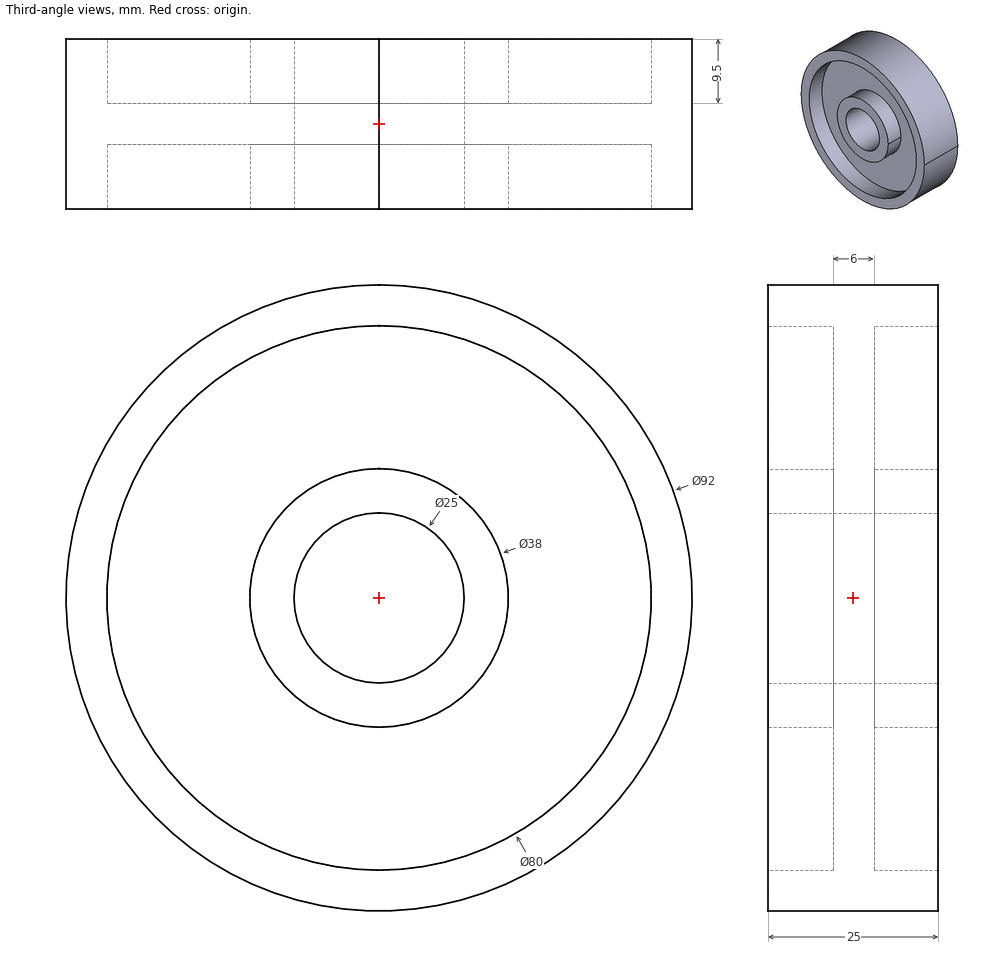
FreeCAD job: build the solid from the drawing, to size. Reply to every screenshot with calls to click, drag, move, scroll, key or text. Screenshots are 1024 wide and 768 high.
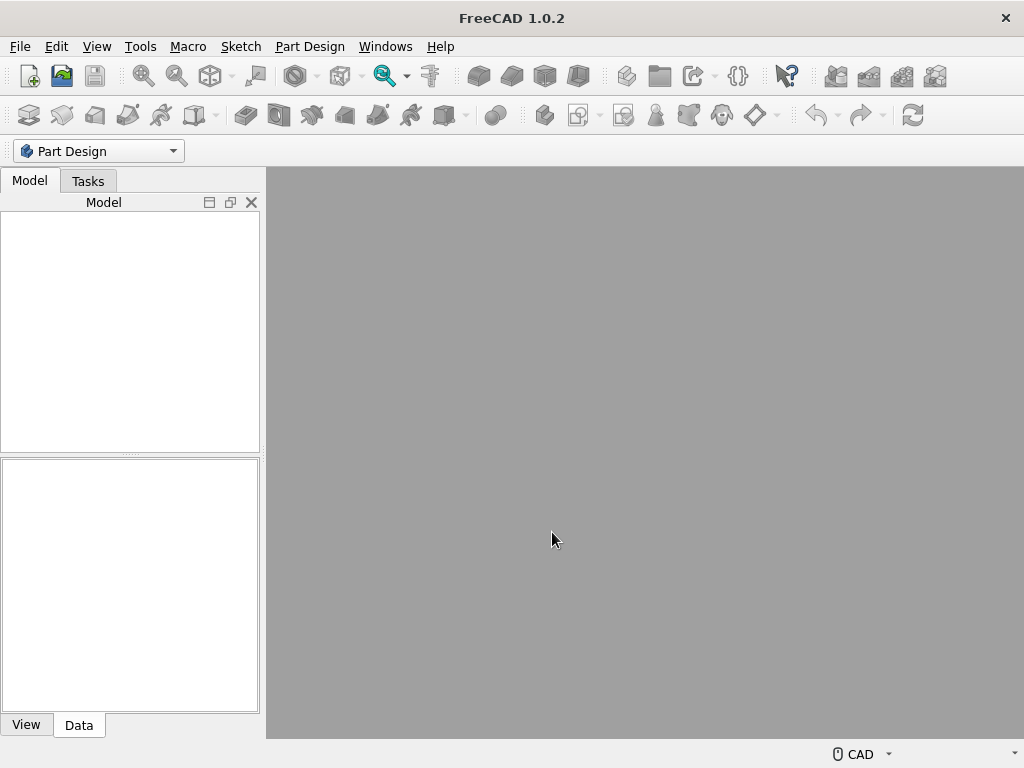
click(29, 76)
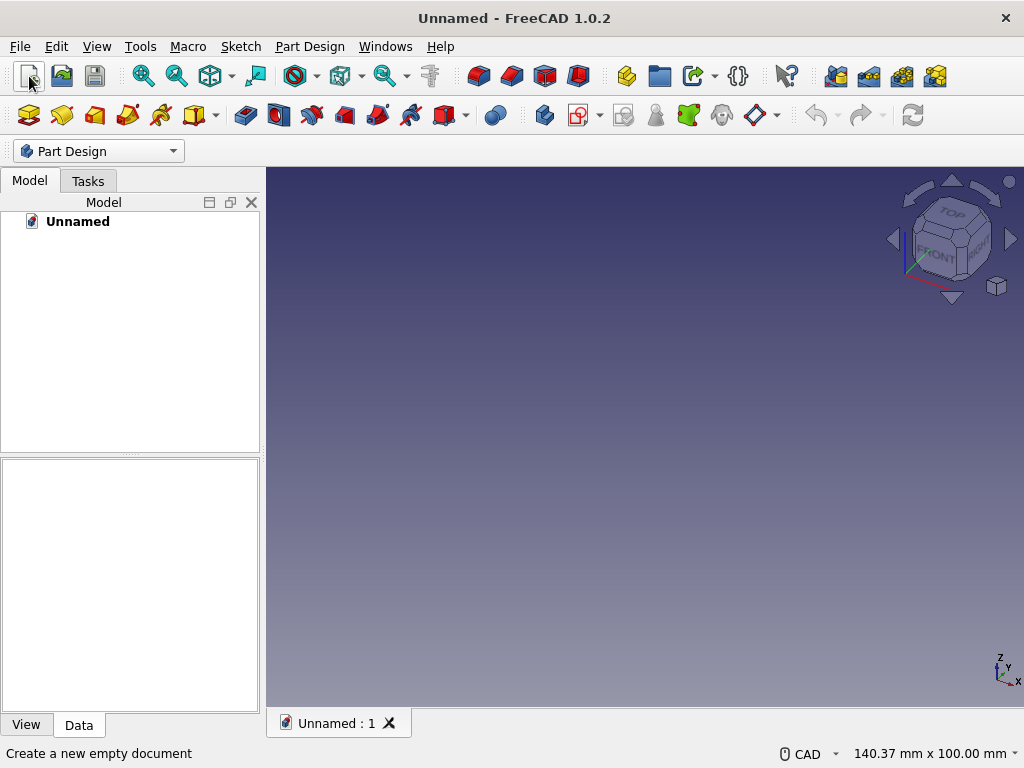
click(578, 116)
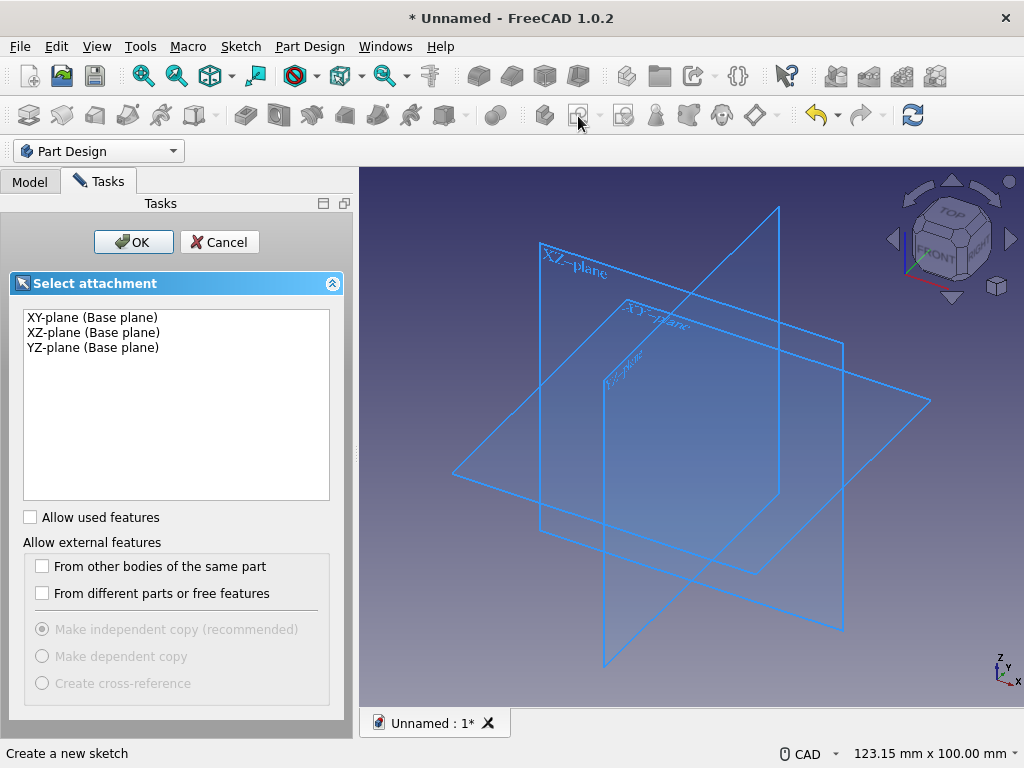
click(84, 332)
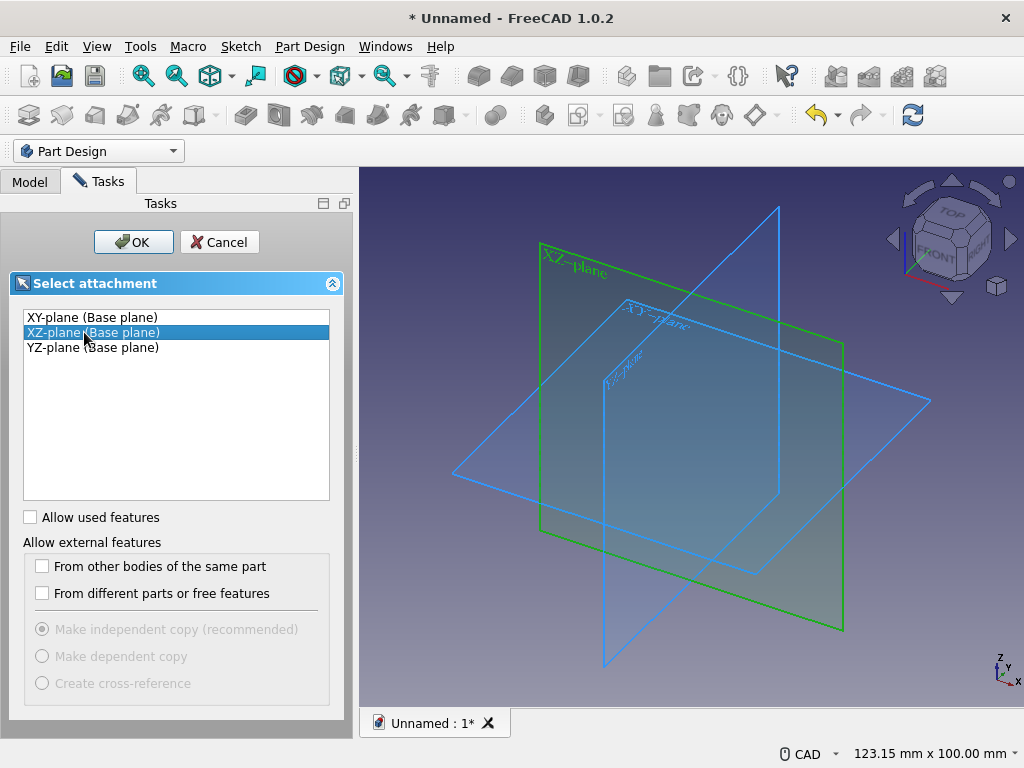
click(134, 242)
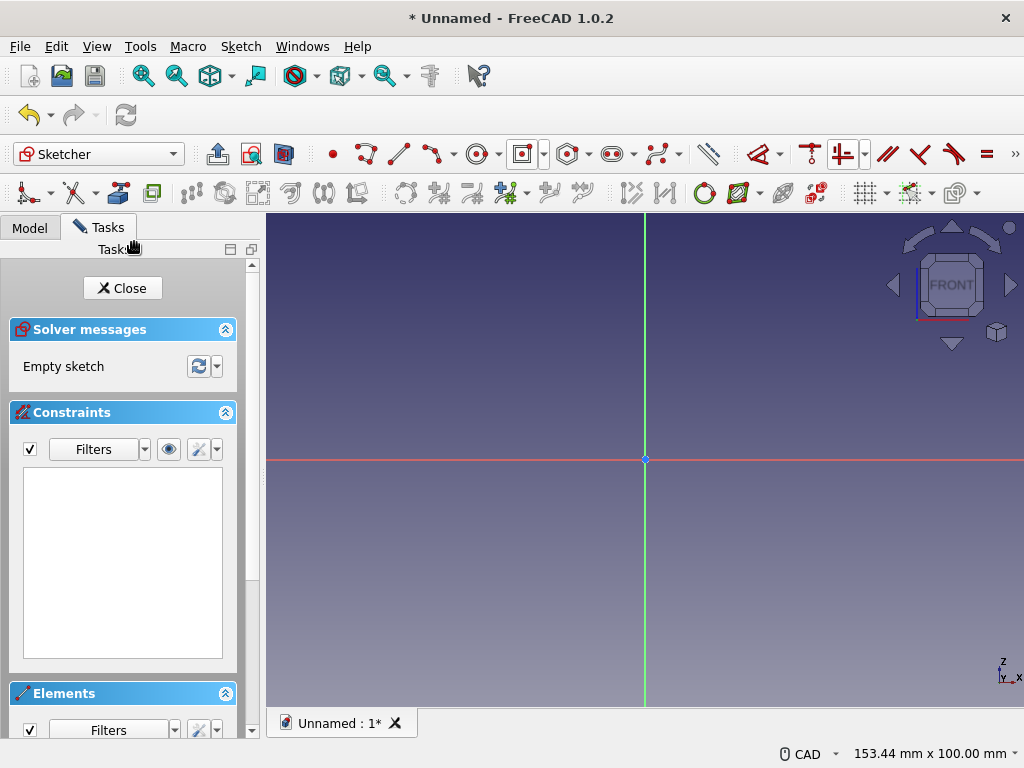
scroll(437, 460, down, 2)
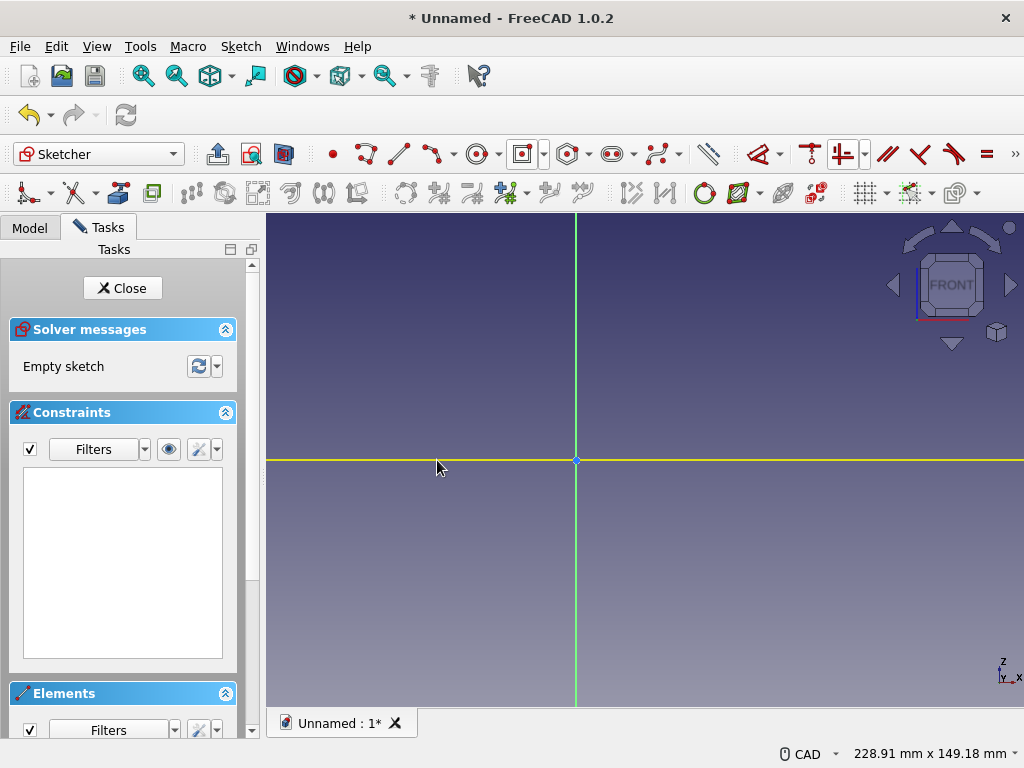
key(g)
key(c)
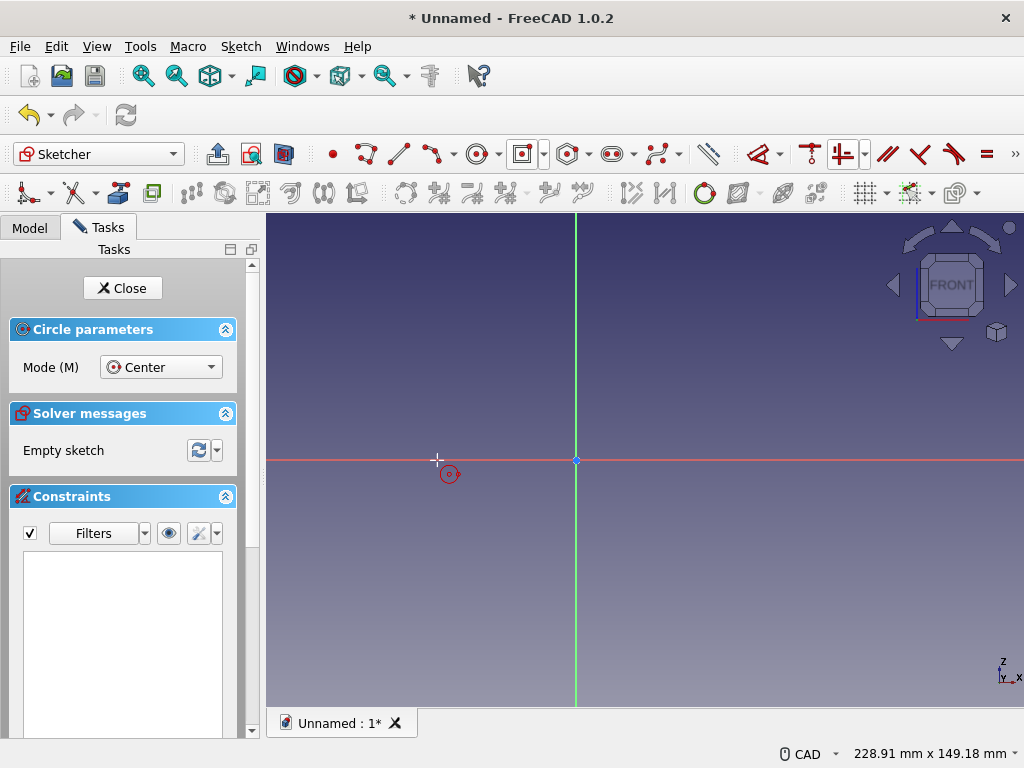
click(577, 460)
move(684, 352)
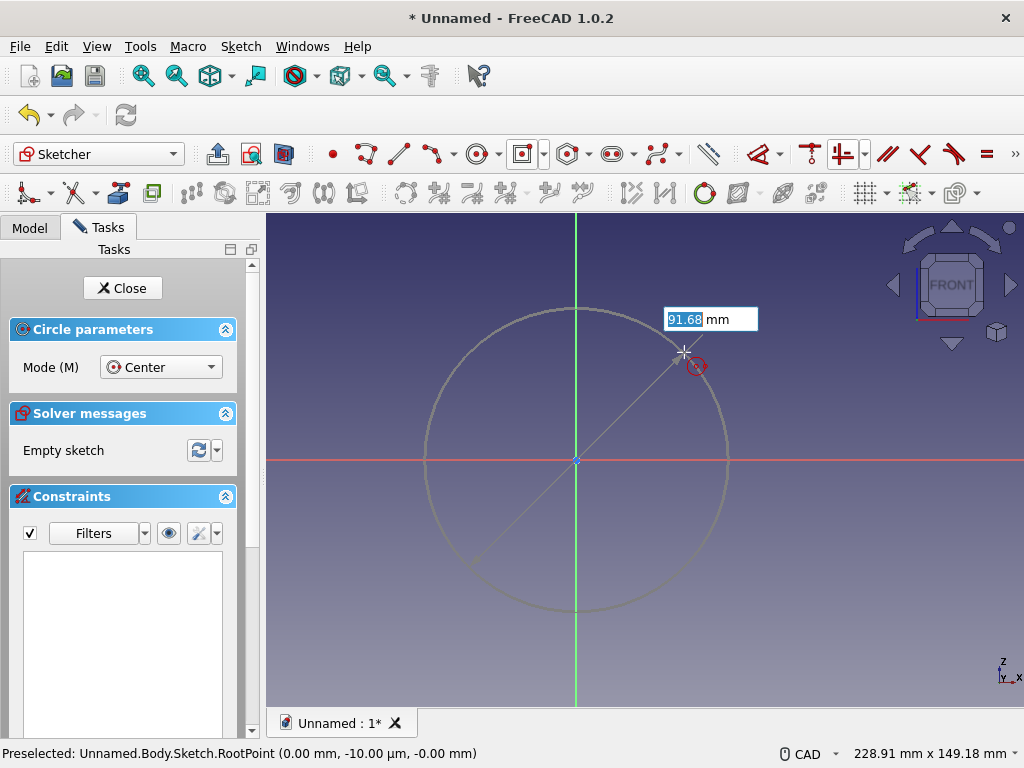
text(92)
key(Return)
key(Escape)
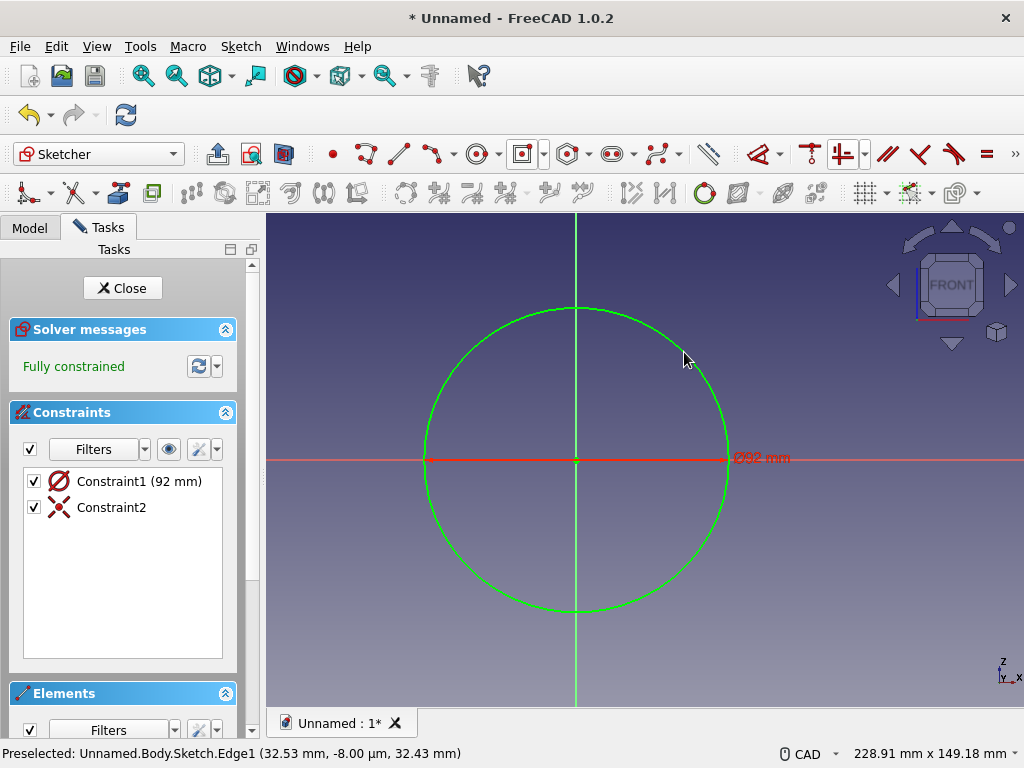
click(123, 288)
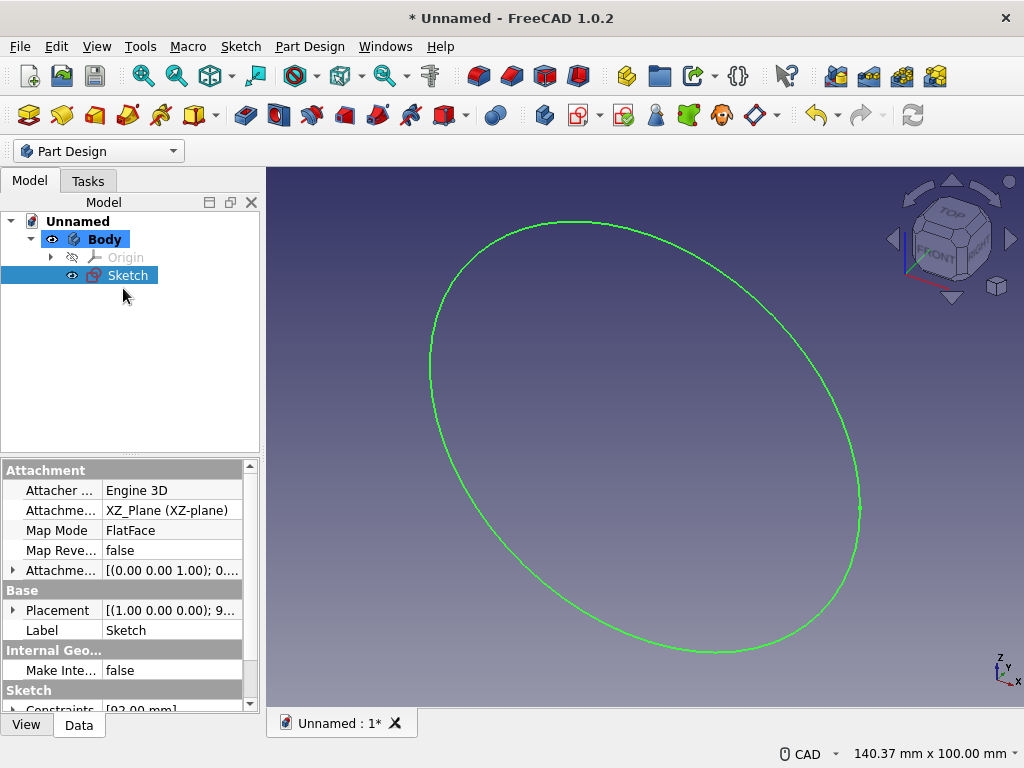
click(29, 116)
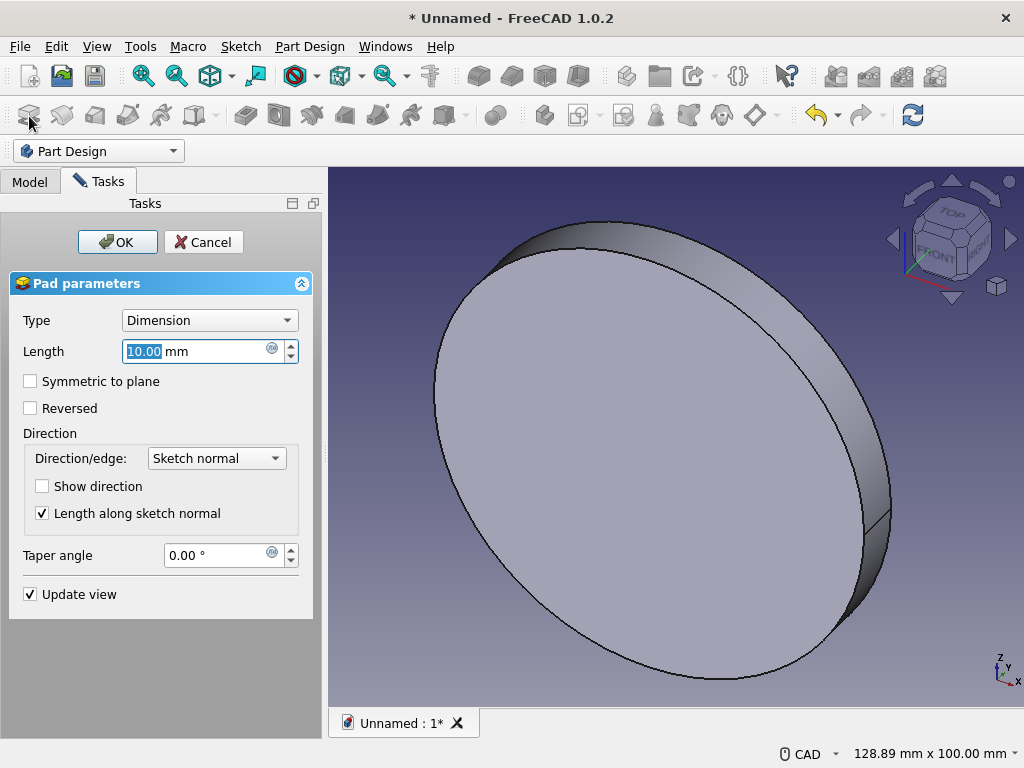
text(6)
key(Tab)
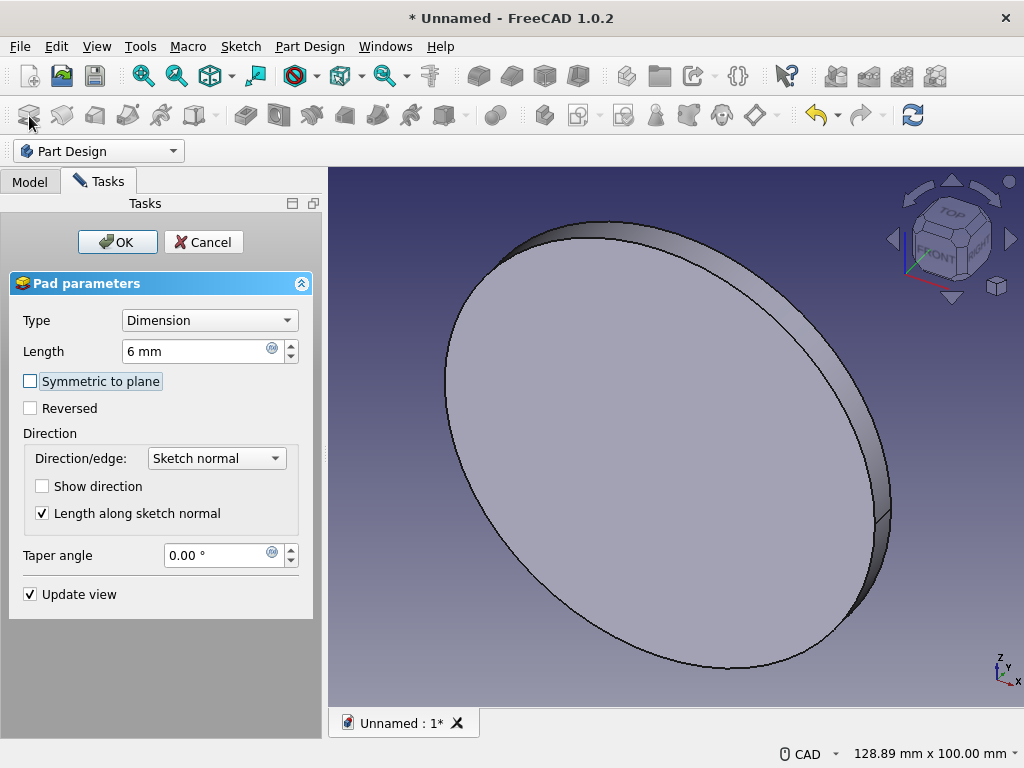
click(31, 381)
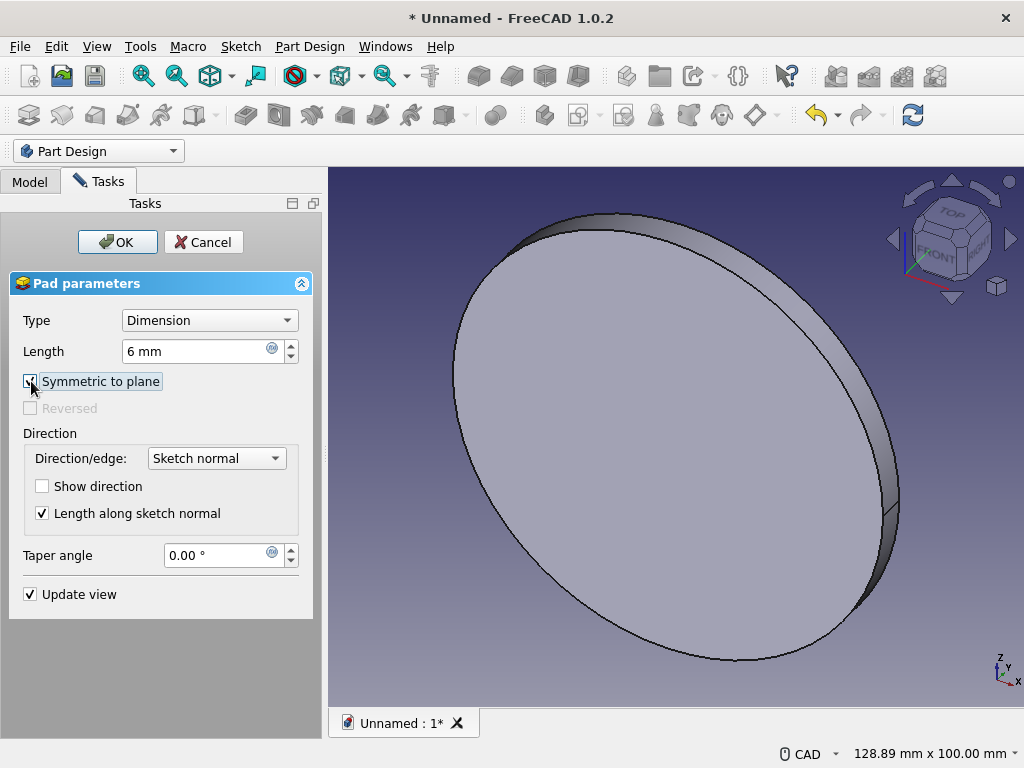
click(118, 242)